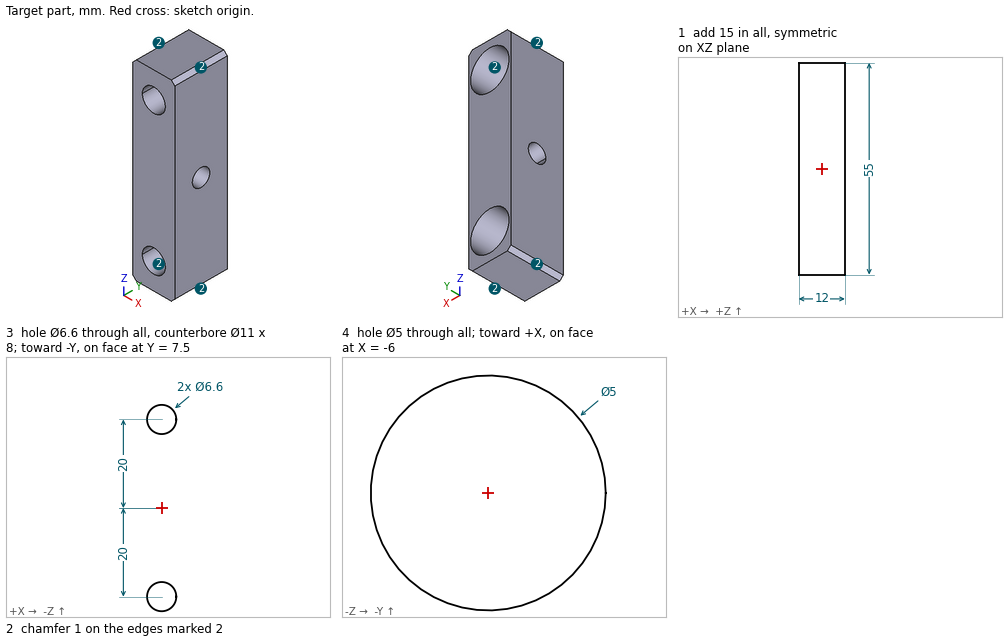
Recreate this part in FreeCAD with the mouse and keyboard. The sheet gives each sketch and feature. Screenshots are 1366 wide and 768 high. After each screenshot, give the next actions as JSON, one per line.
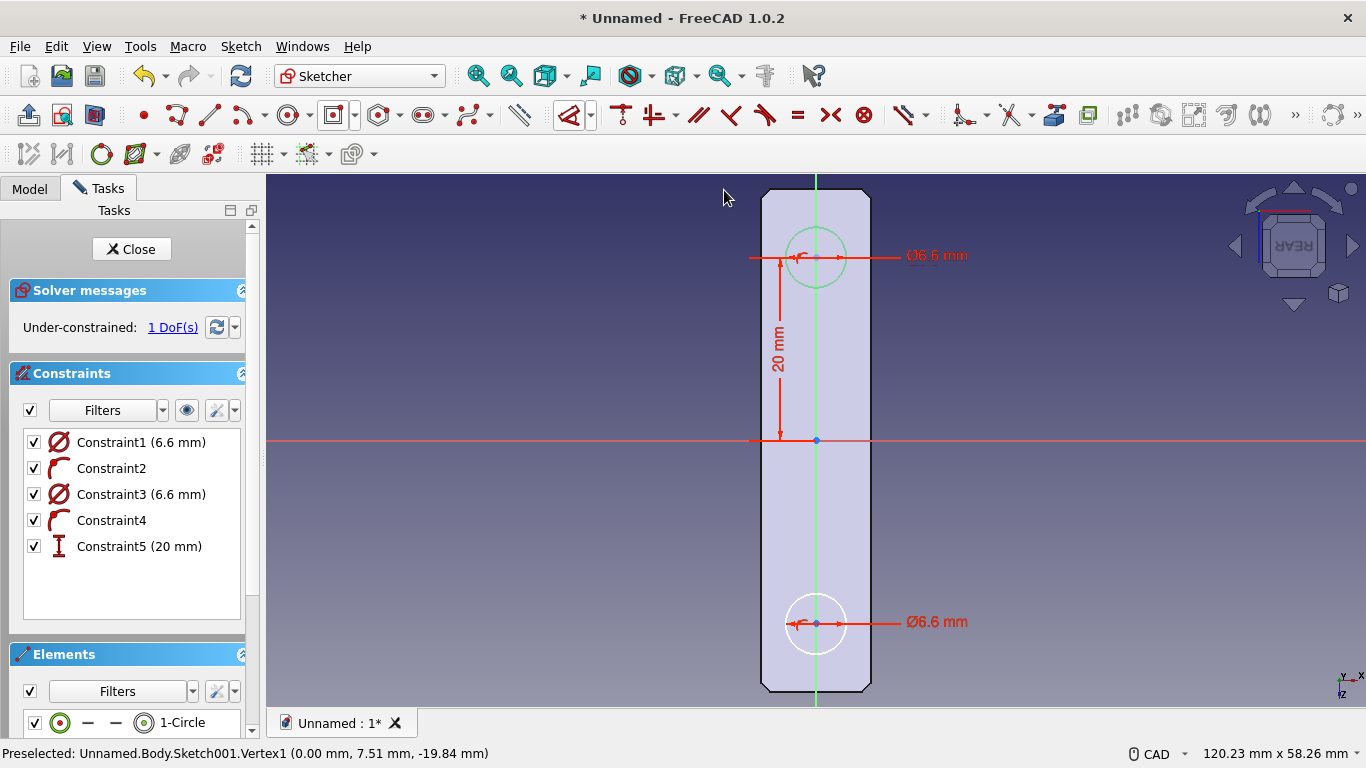
{"action": "left_click", "coordinate": [816, 624]}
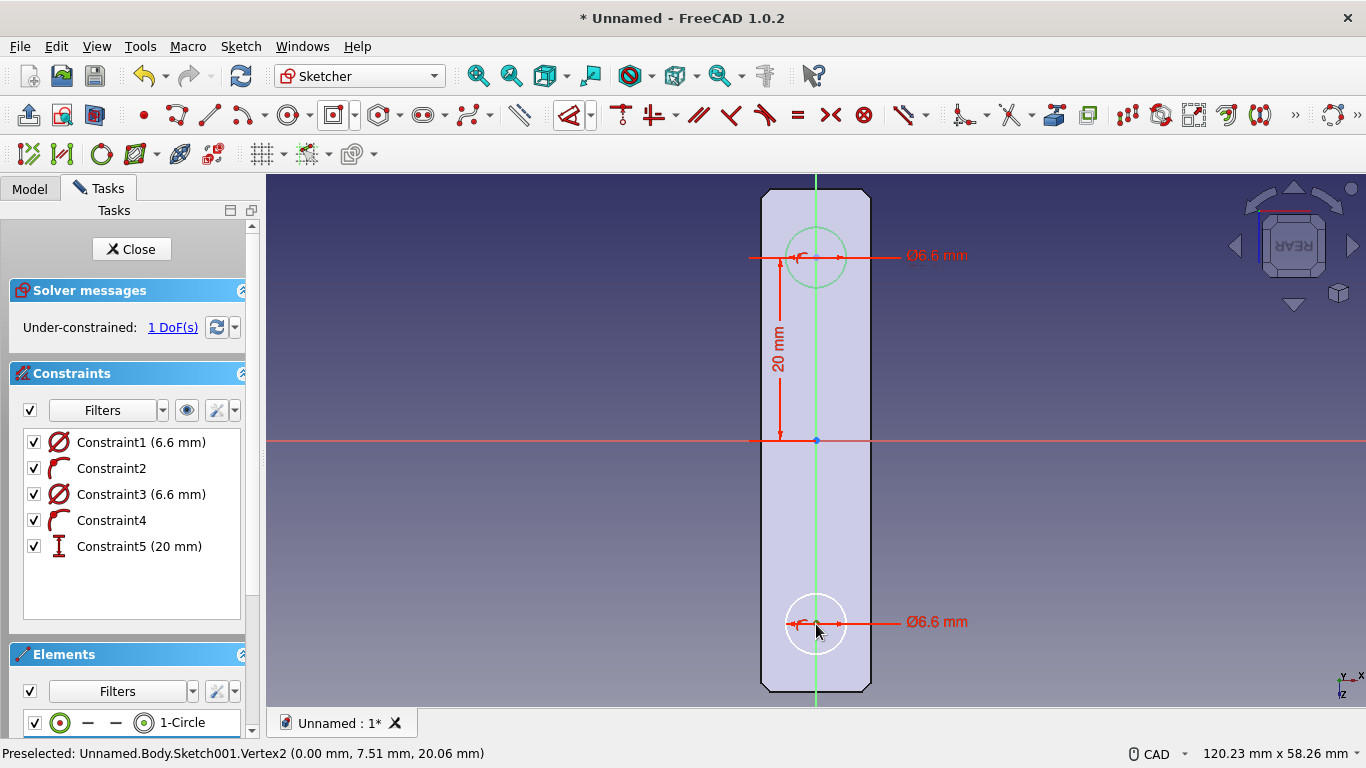
{"action": "left_click", "coordinate": [590, 116]}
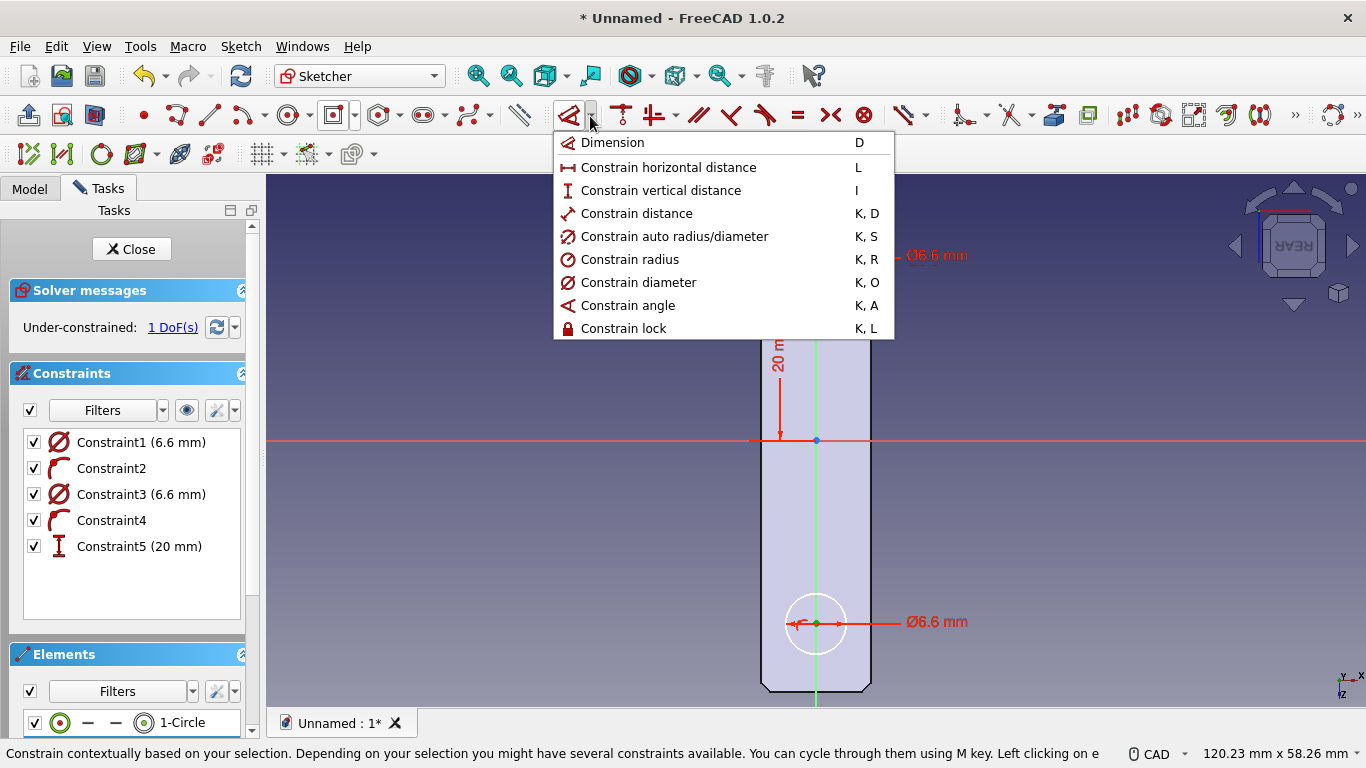
{"action": "left_click", "coordinate": [724, 190]}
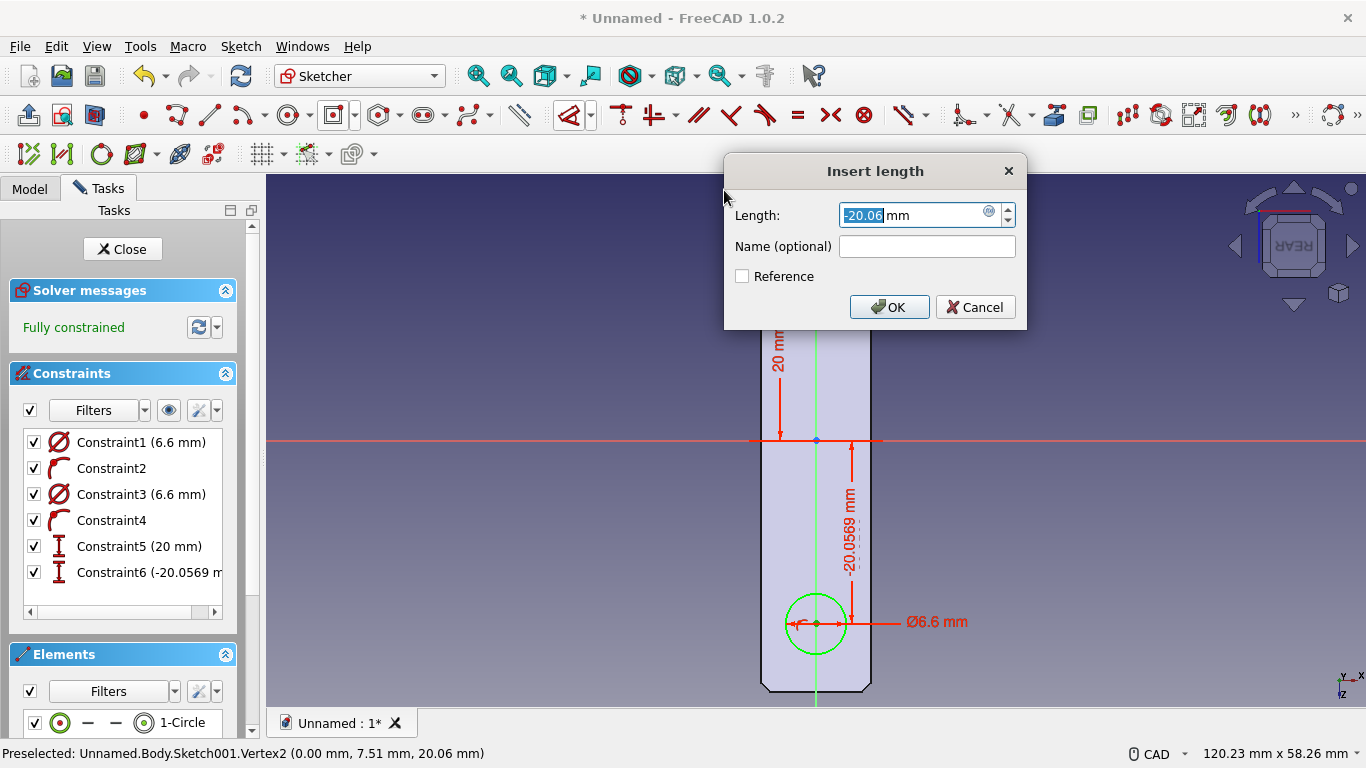
{"action": "type", "text": "-20"}
{"action": "key", "text": "Return"}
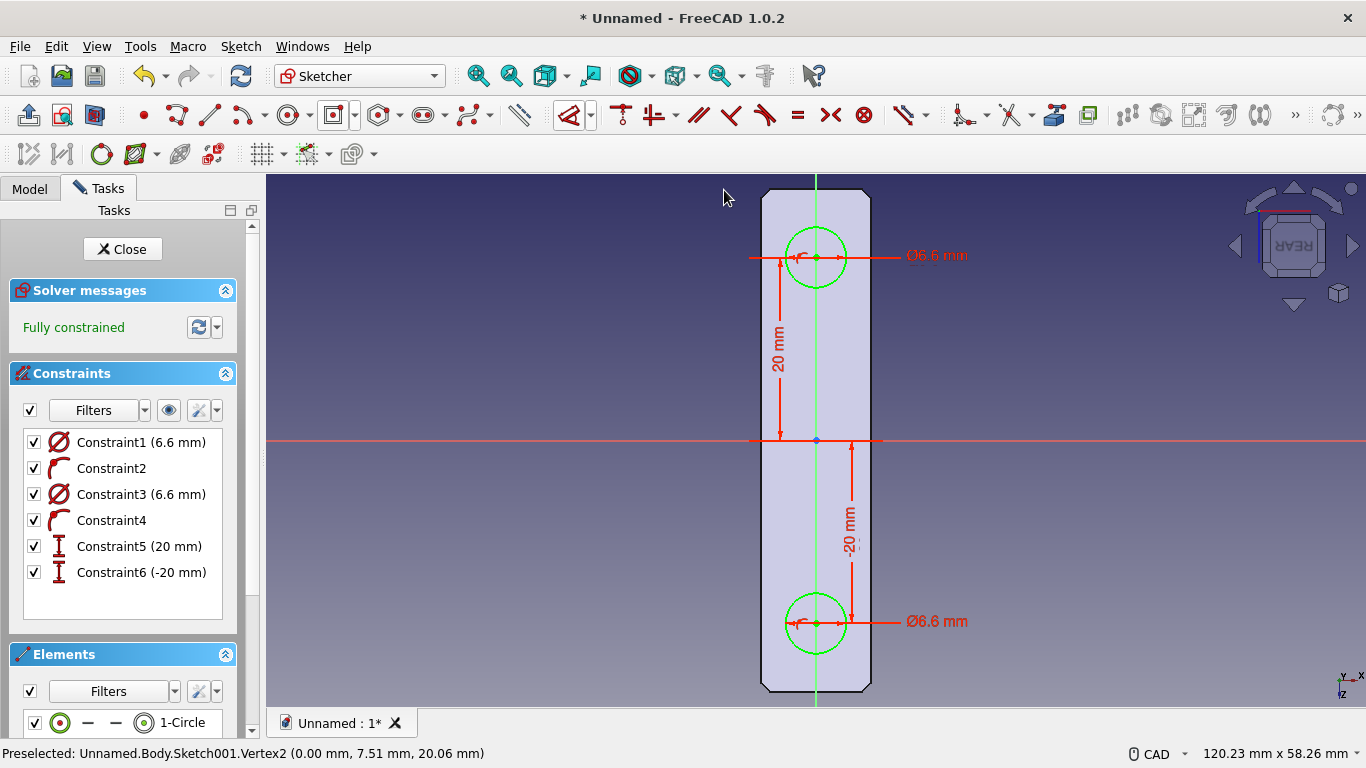
{"action": "left_click", "coordinate": [123, 249]}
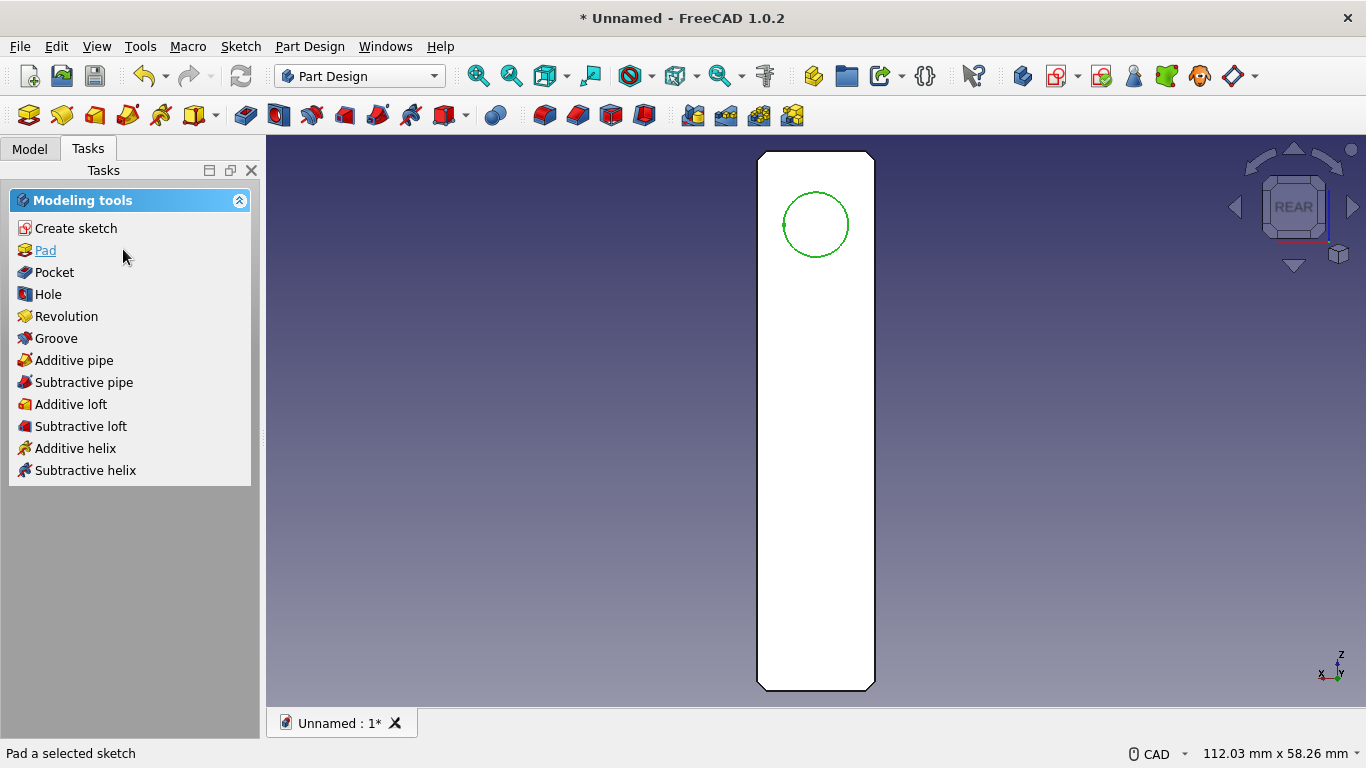
{"action": "left_click", "coordinate": [279, 116]}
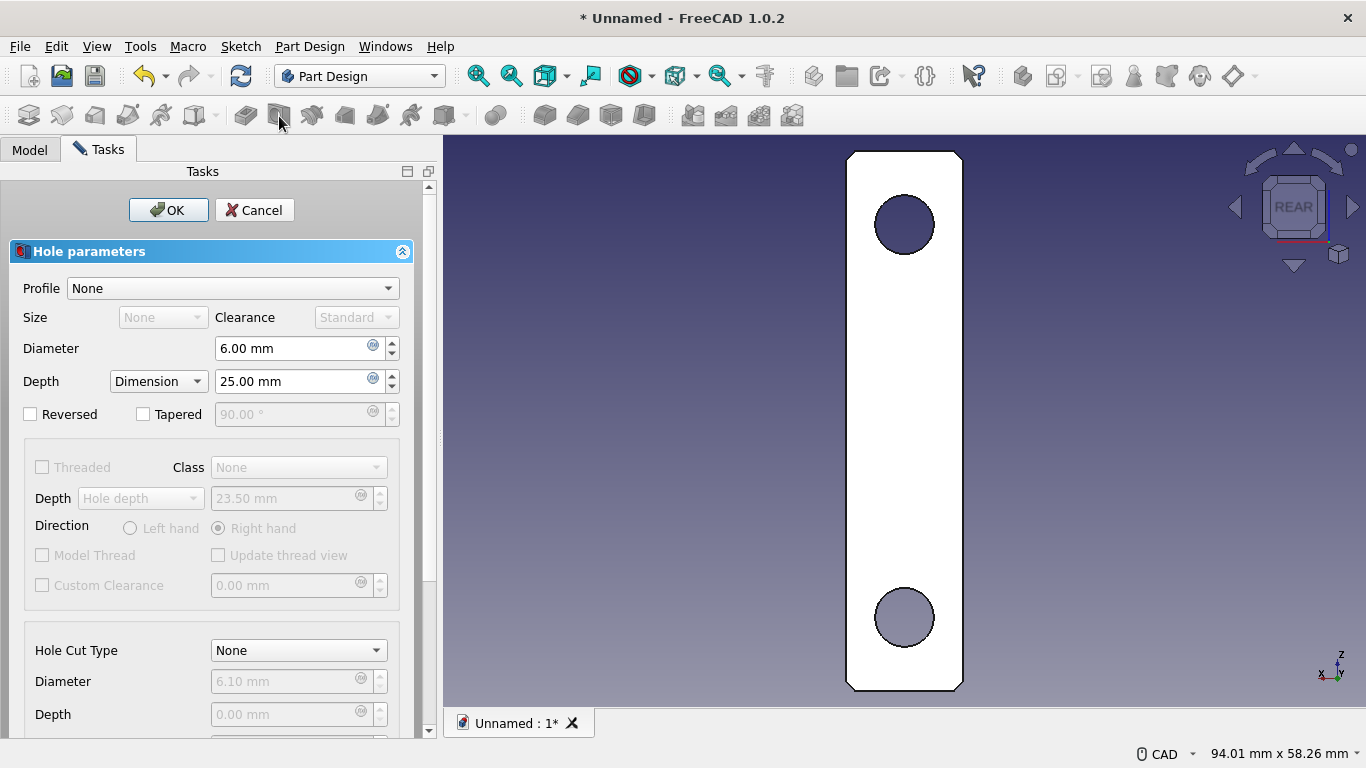
{"action": "triple_click", "coordinate": [300, 348]}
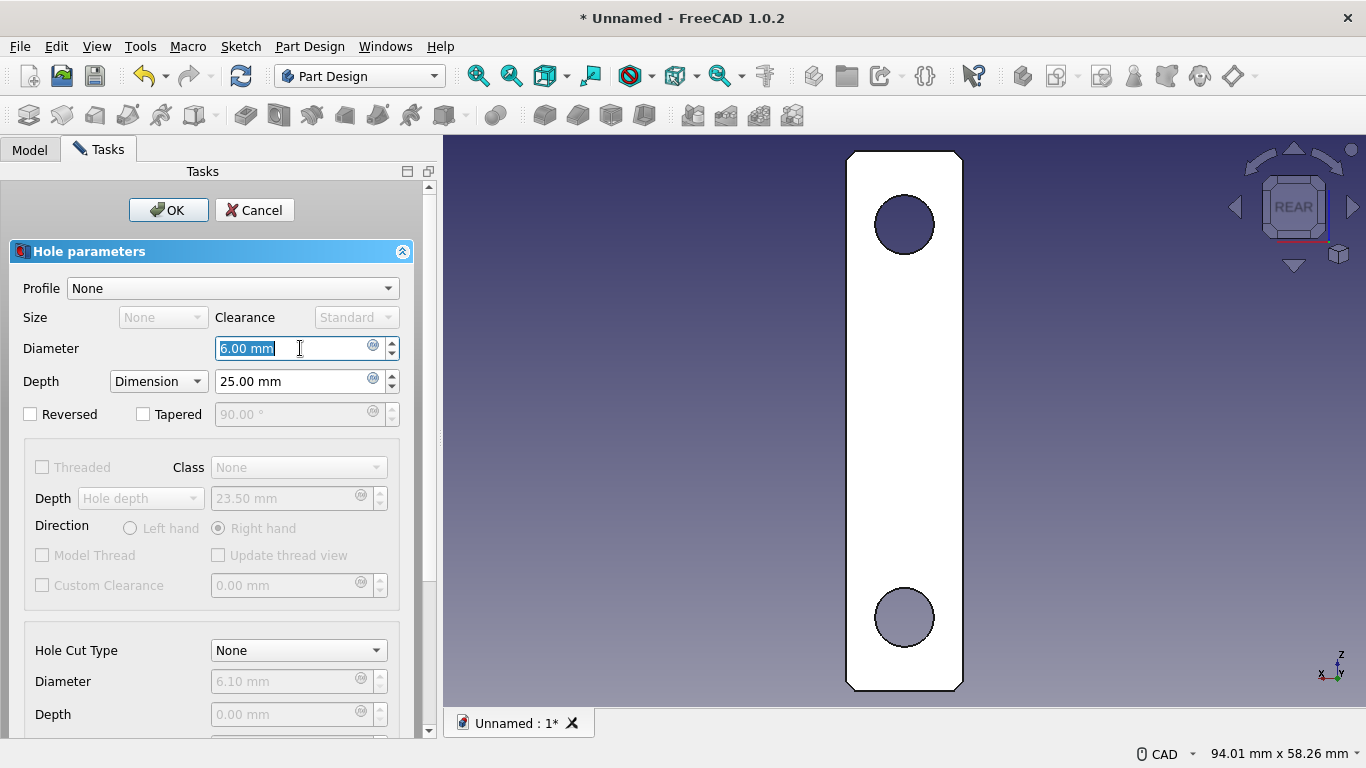
{"action": "type", "text": "6.6"}
{"action": "key", "text": "Tab"}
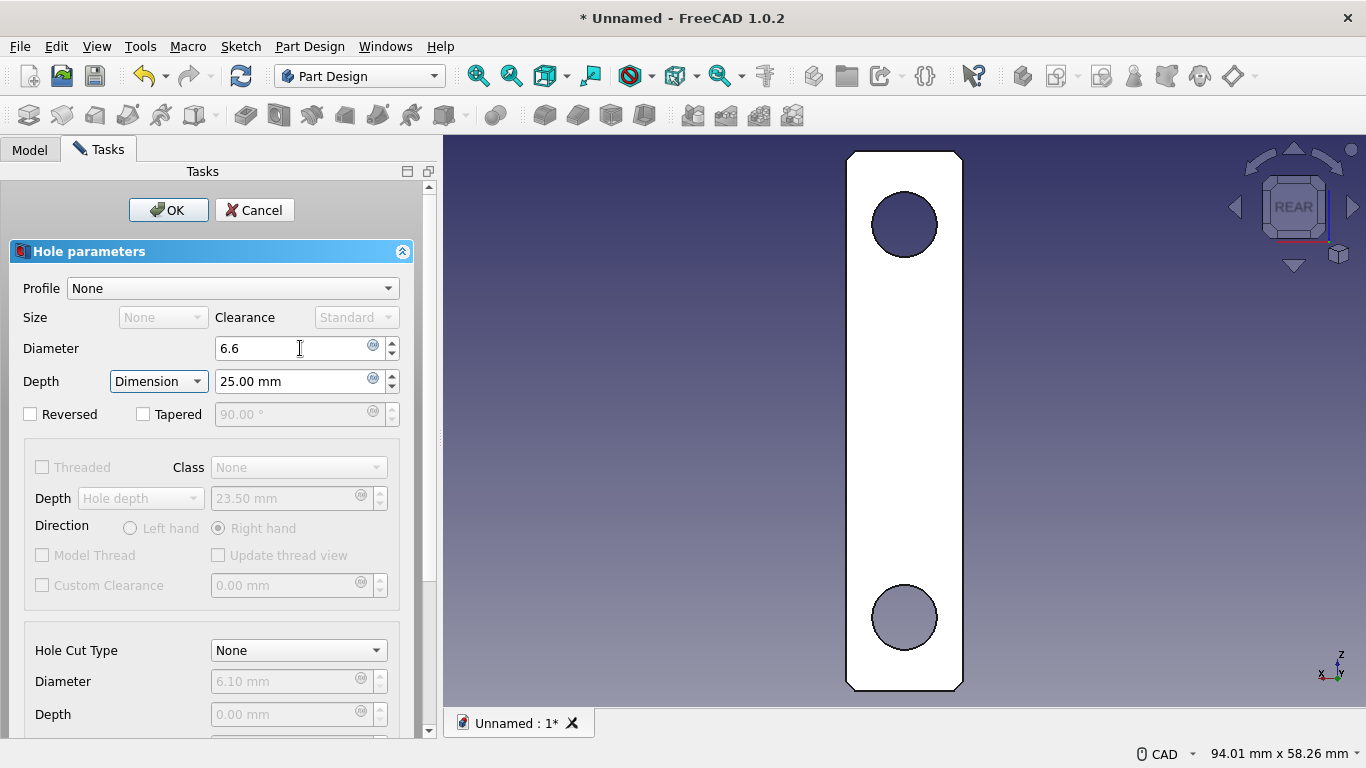
{"action": "left_click", "coordinate": [160, 382]}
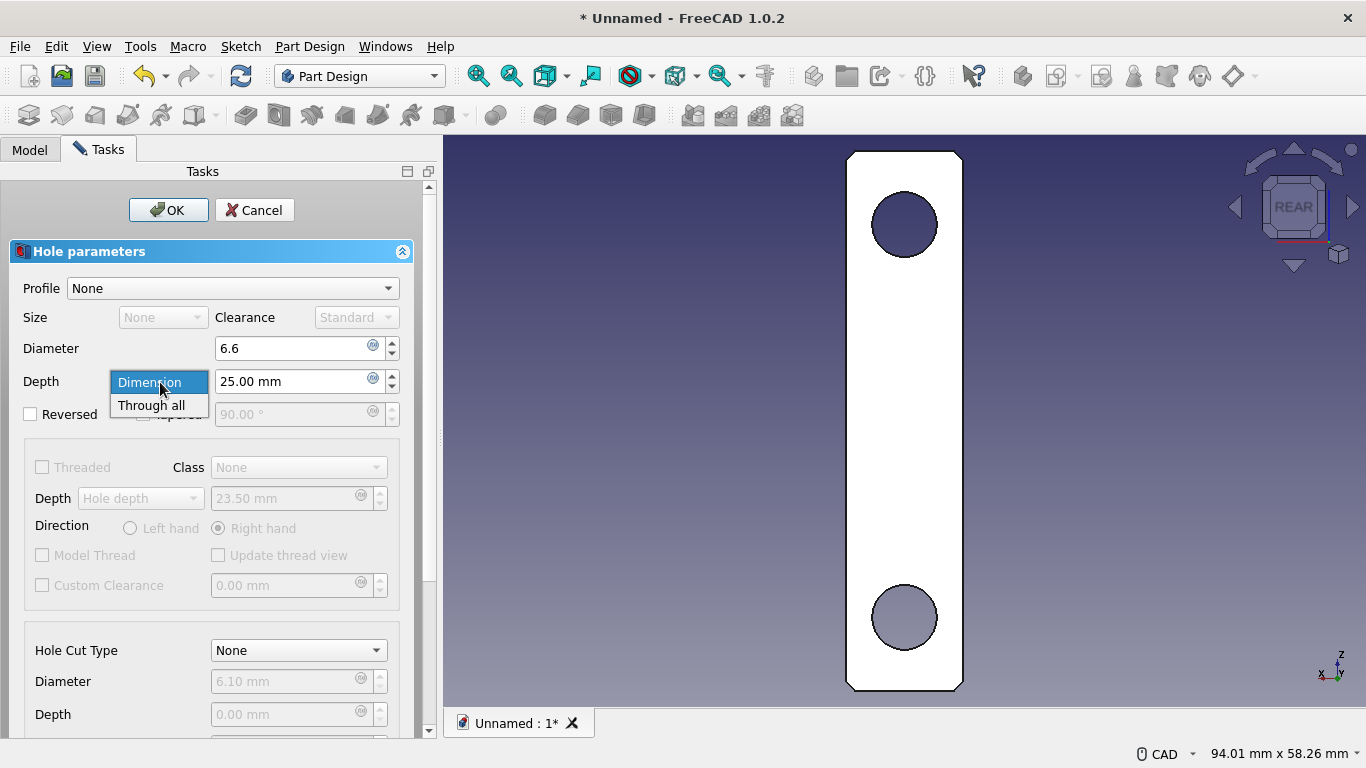
{"action": "left_click", "coordinate": [158, 406]}